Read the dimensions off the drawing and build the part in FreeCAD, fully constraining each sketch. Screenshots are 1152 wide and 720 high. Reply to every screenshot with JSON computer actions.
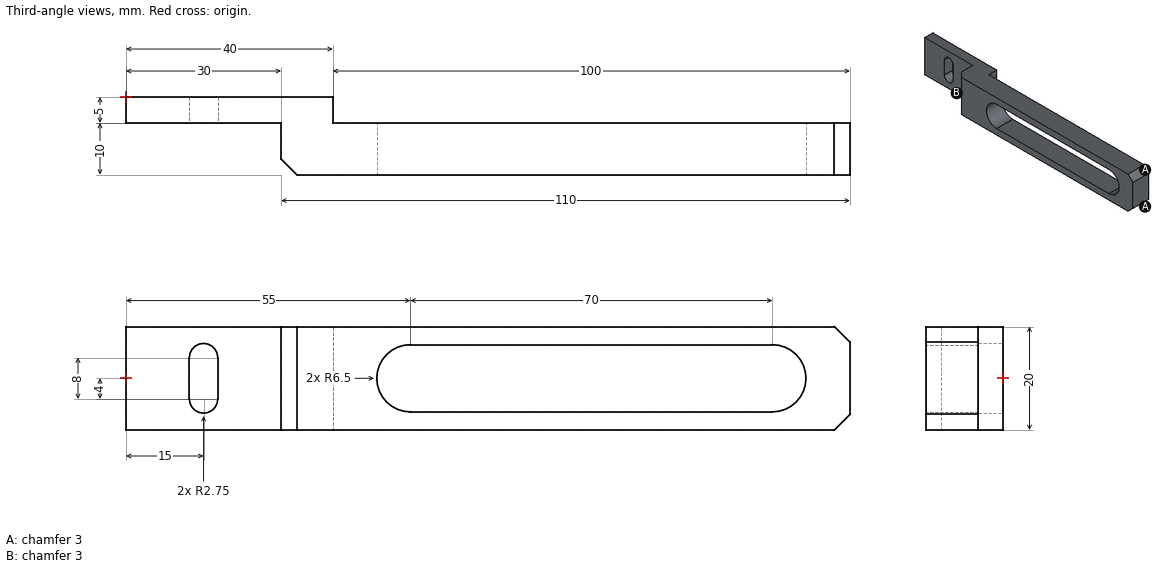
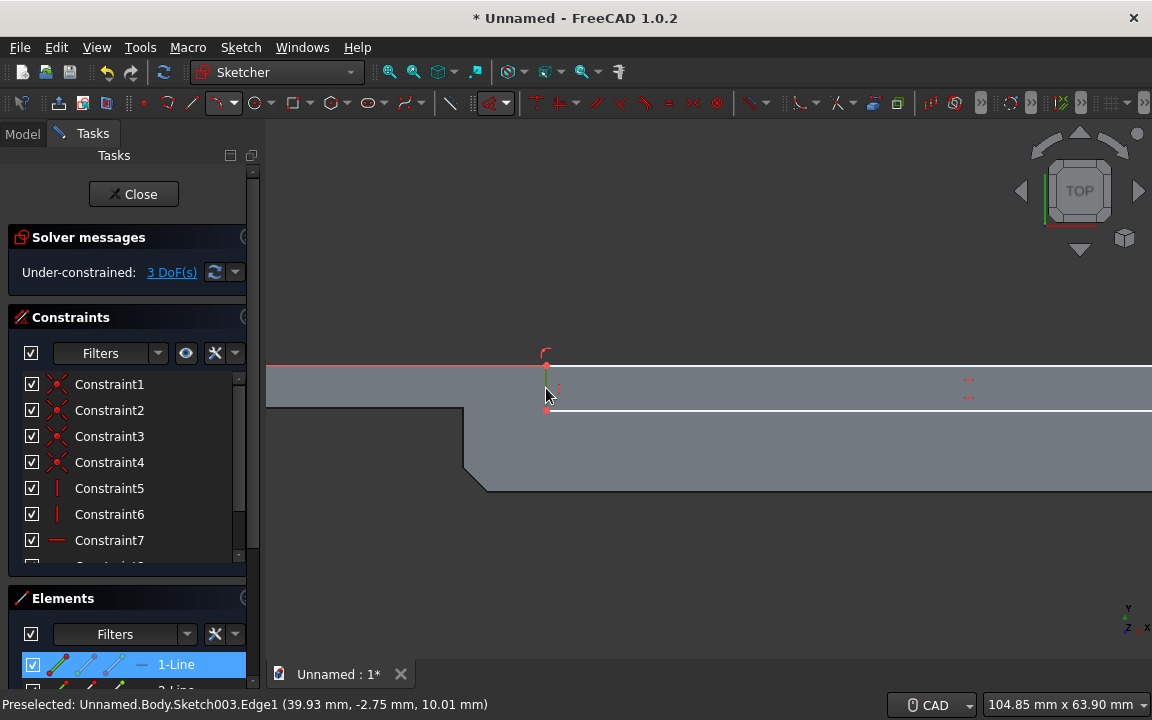
{"action": "key", "text": "i"}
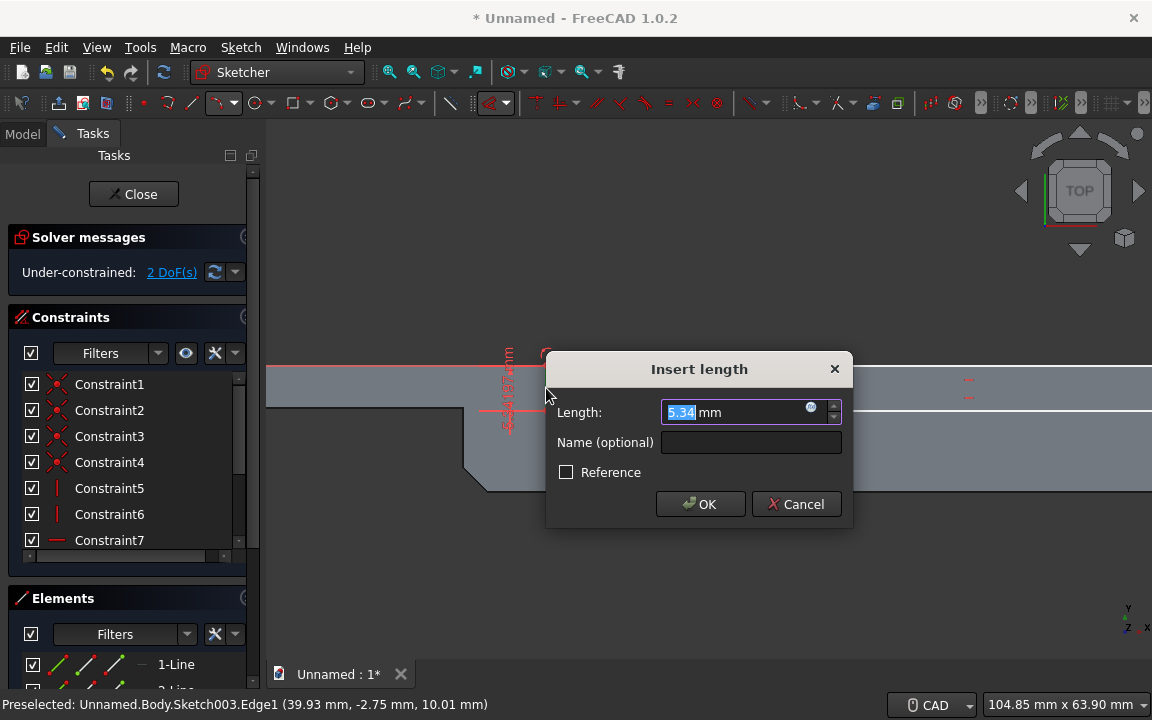
{"action": "type", "text": "5"}
{"action": "key", "text": "Return"}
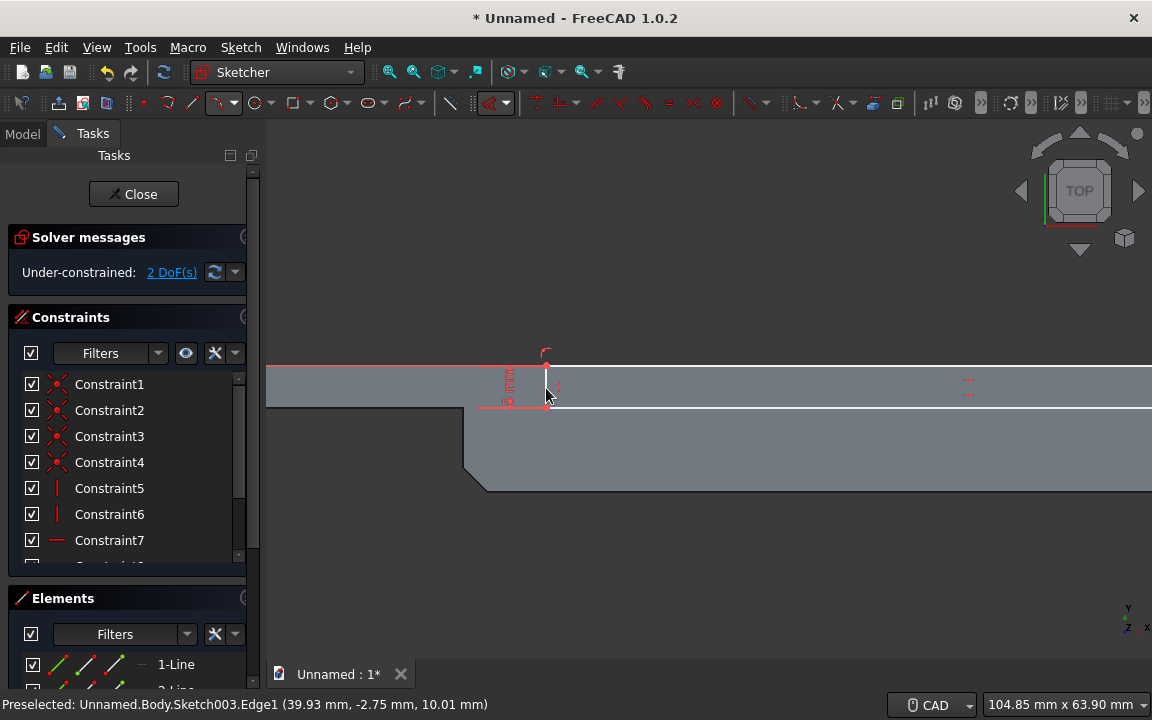
{"action": "left_click", "coordinate": [800, 408]}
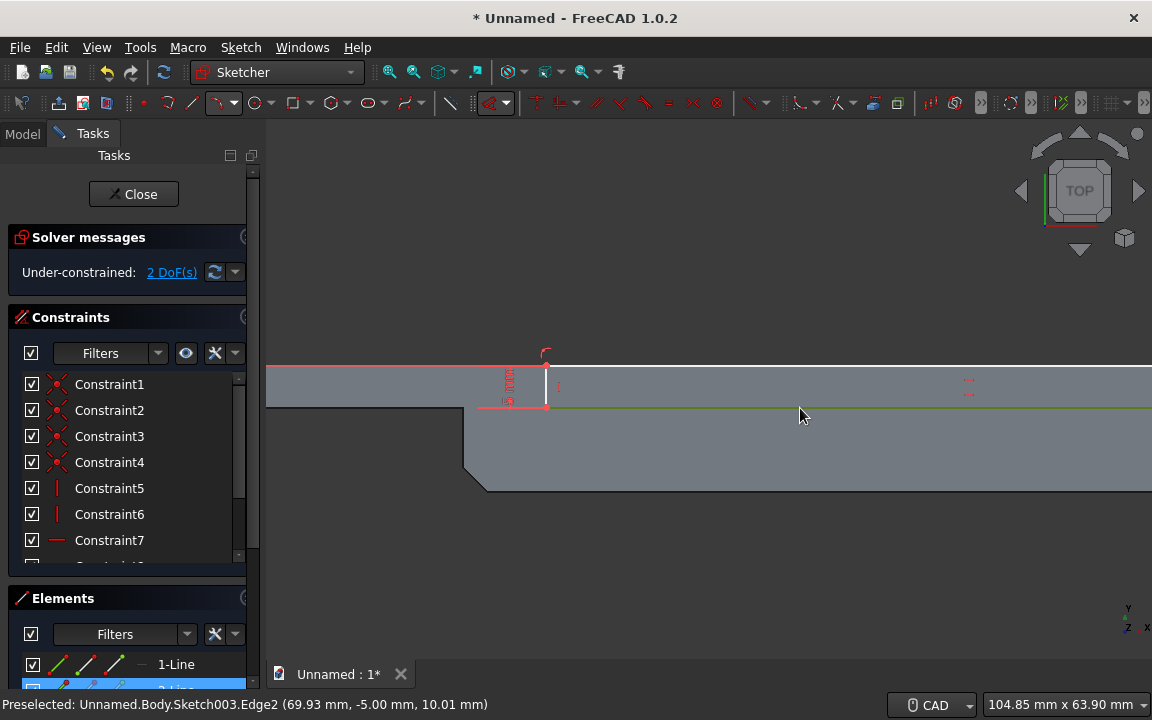
{"action": "left_click", "coordinate": [508, 104]}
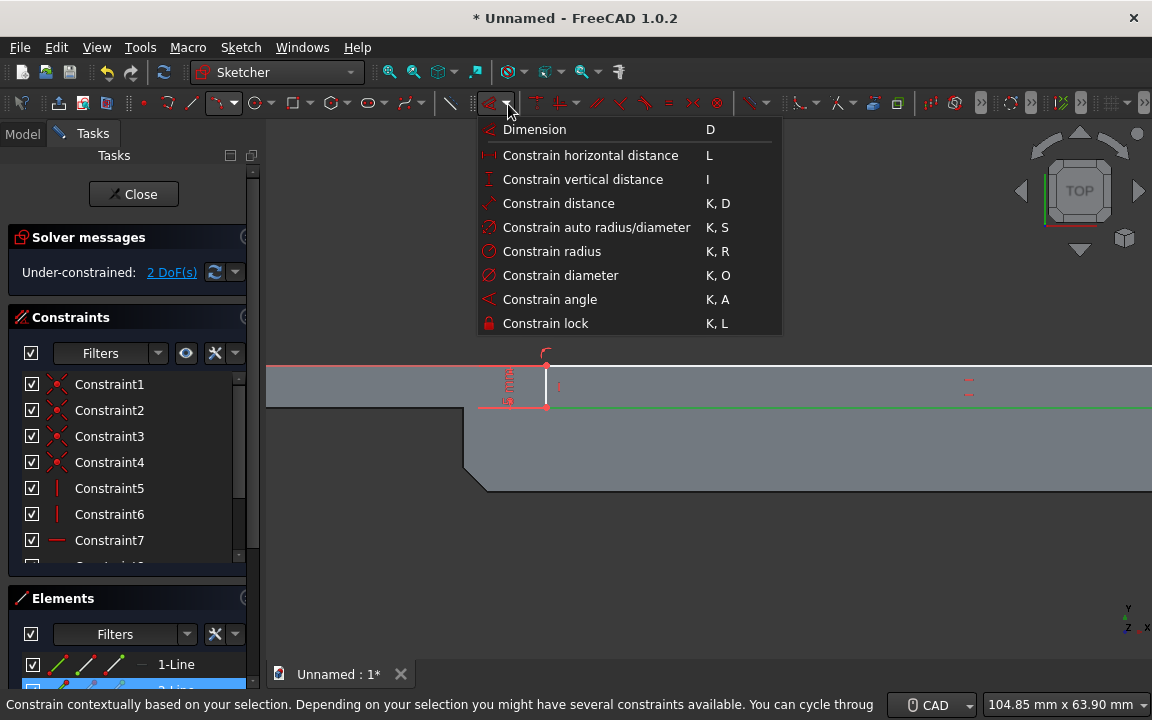
{"action": "left_click", "coordinate": [630, 155]}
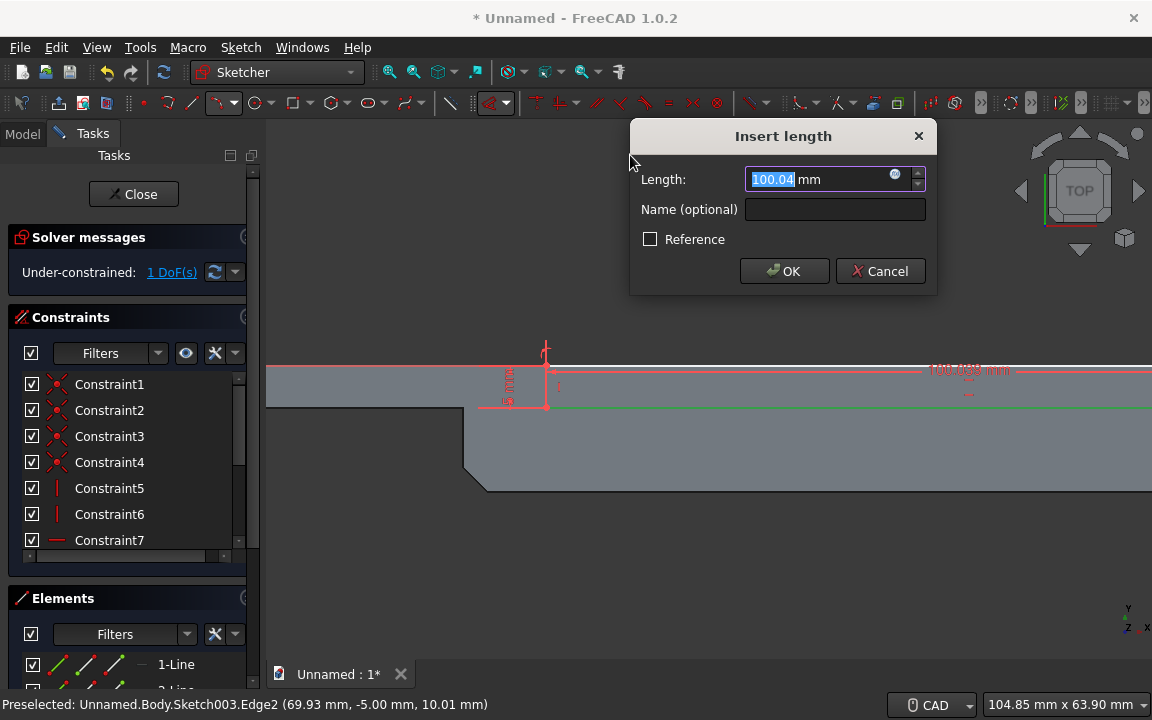
{"action": "type", "text": "100"}
{"action": "key", "text": "Return"}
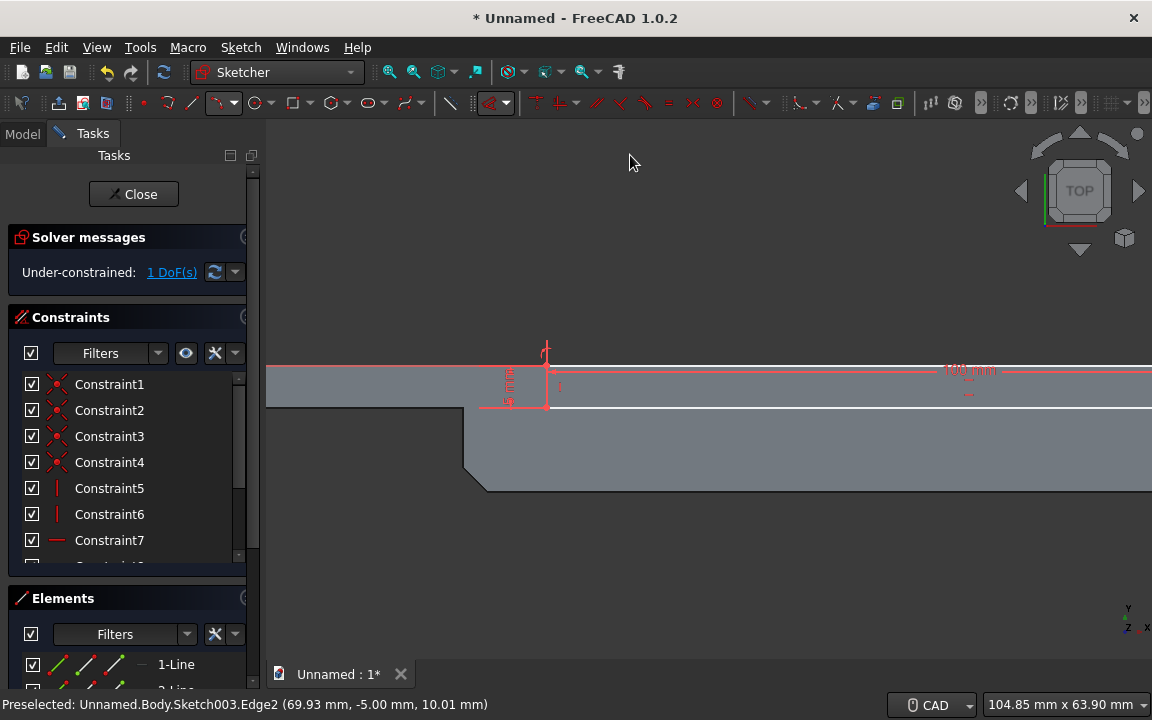
{"action": "left_click", "coordinate": [547, 366]}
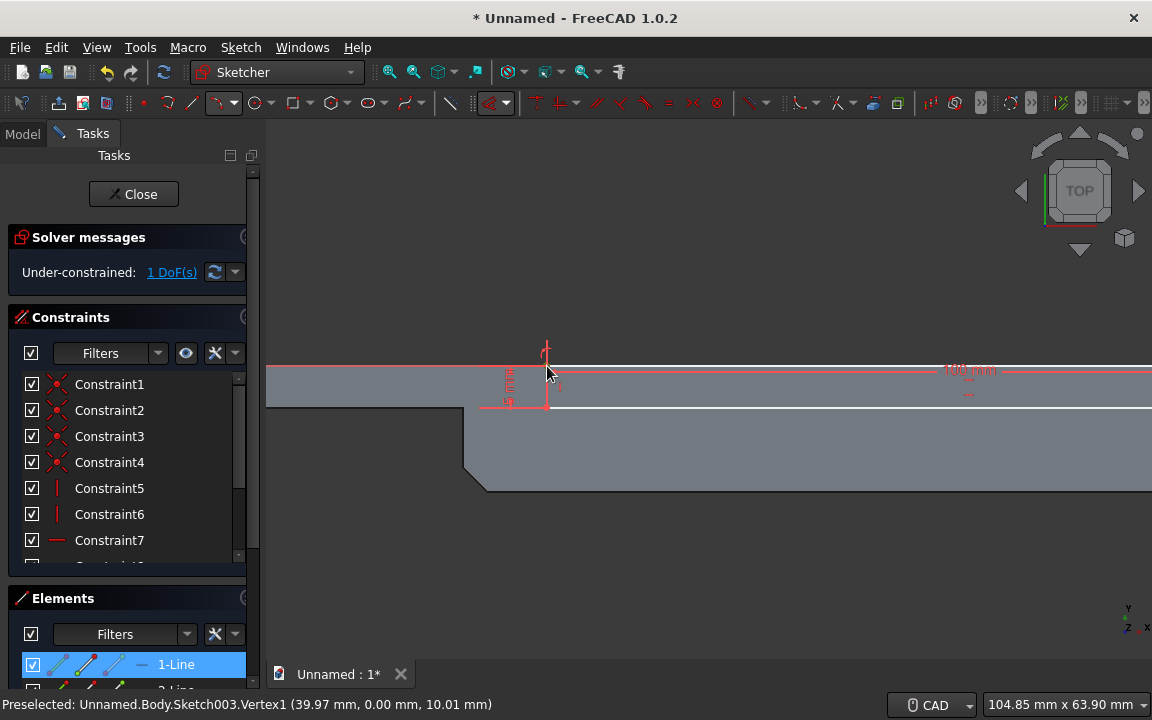
{"action": "key", "text": "l"}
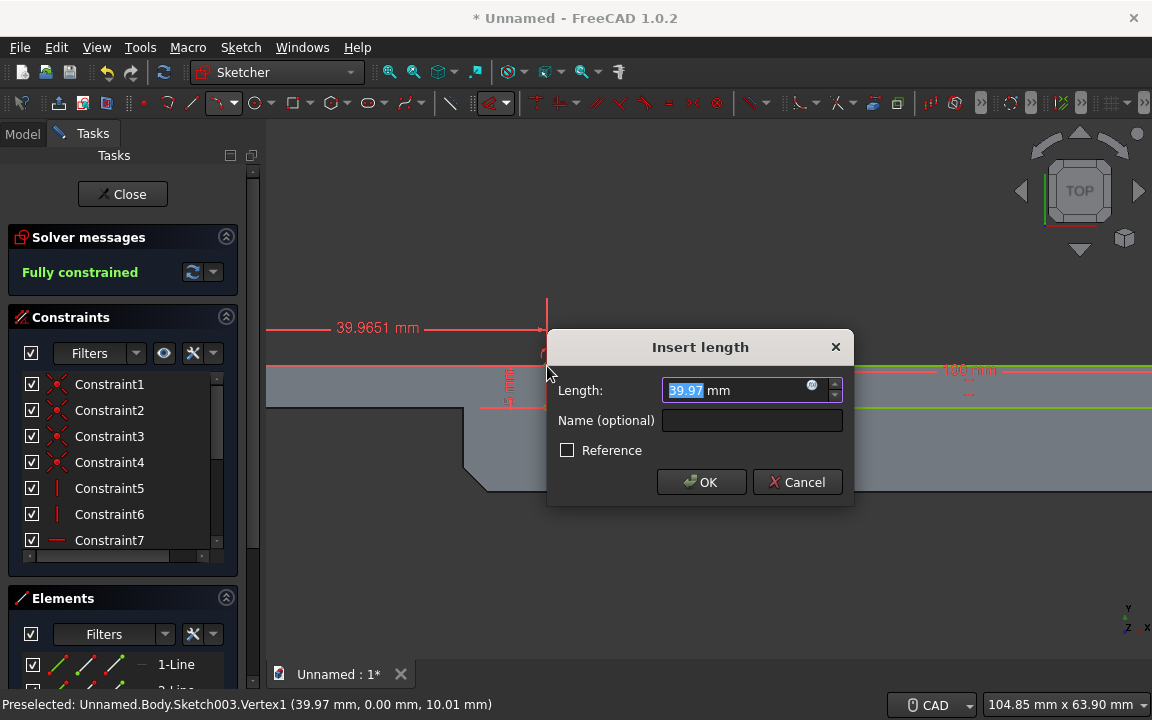
{"action": "type", "text": "40"}
{"action": "key", "text": "Return"}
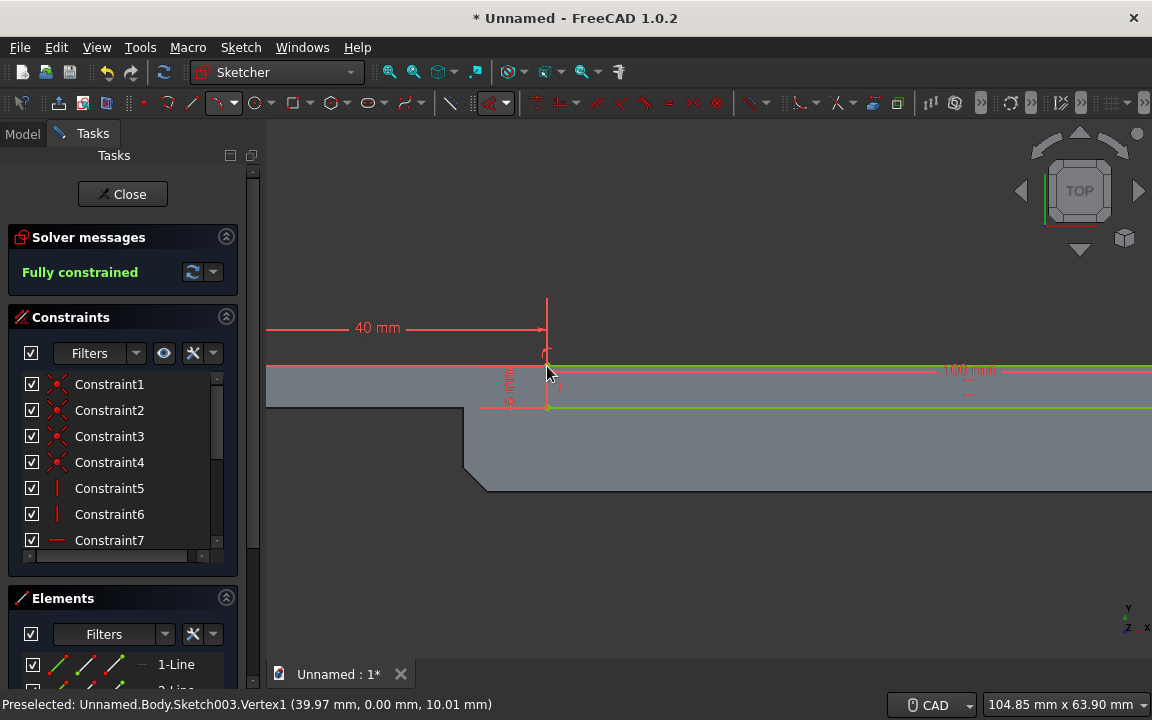
{"action": "left_click", "coordinate": [123, 194]}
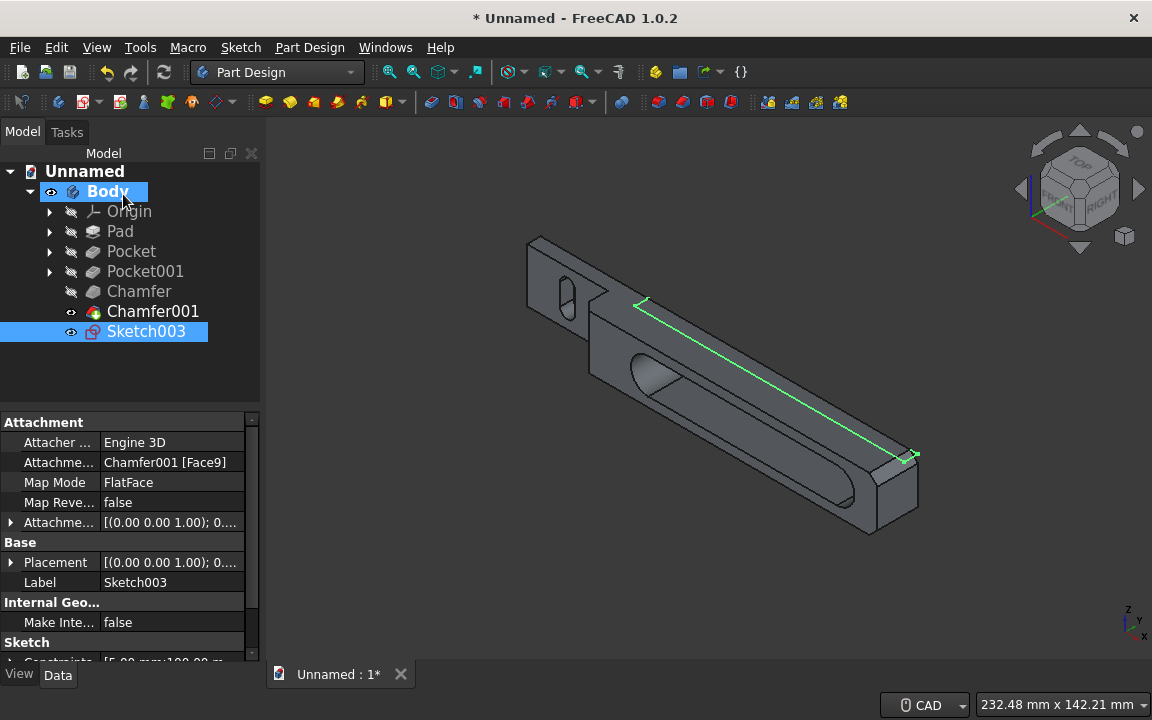
{"action": "left_click", "coordinate": [432, 102]}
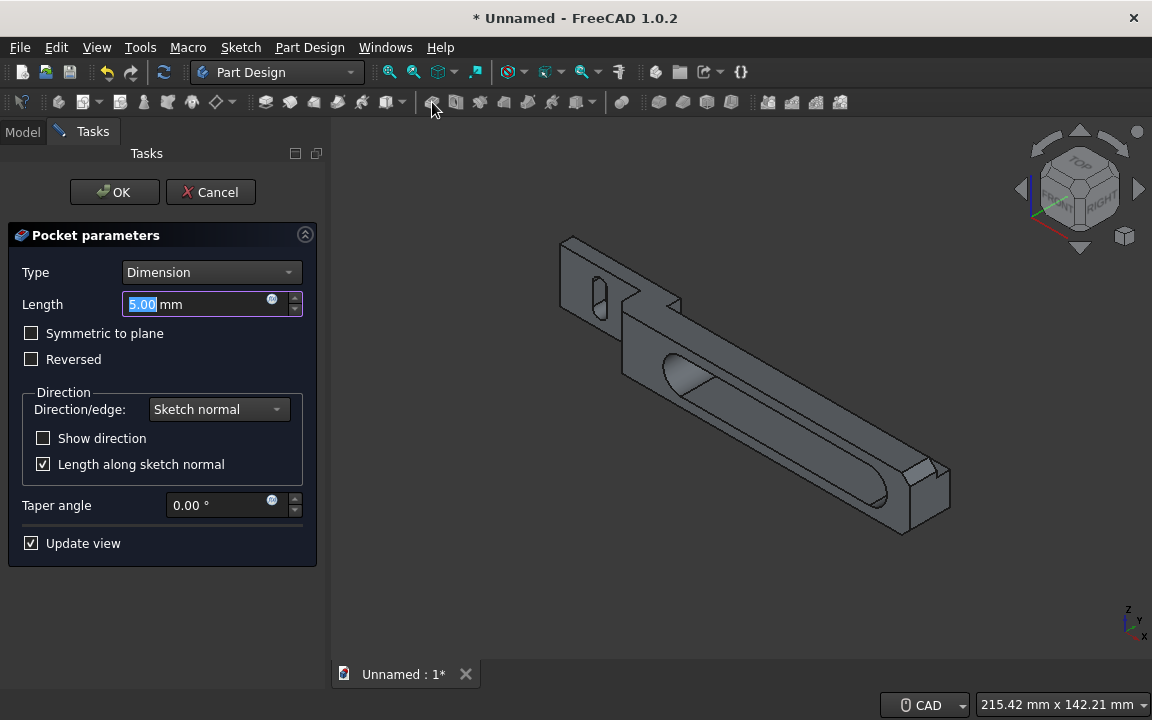
{"action": "left_click", "coordinate": [212, 272]}